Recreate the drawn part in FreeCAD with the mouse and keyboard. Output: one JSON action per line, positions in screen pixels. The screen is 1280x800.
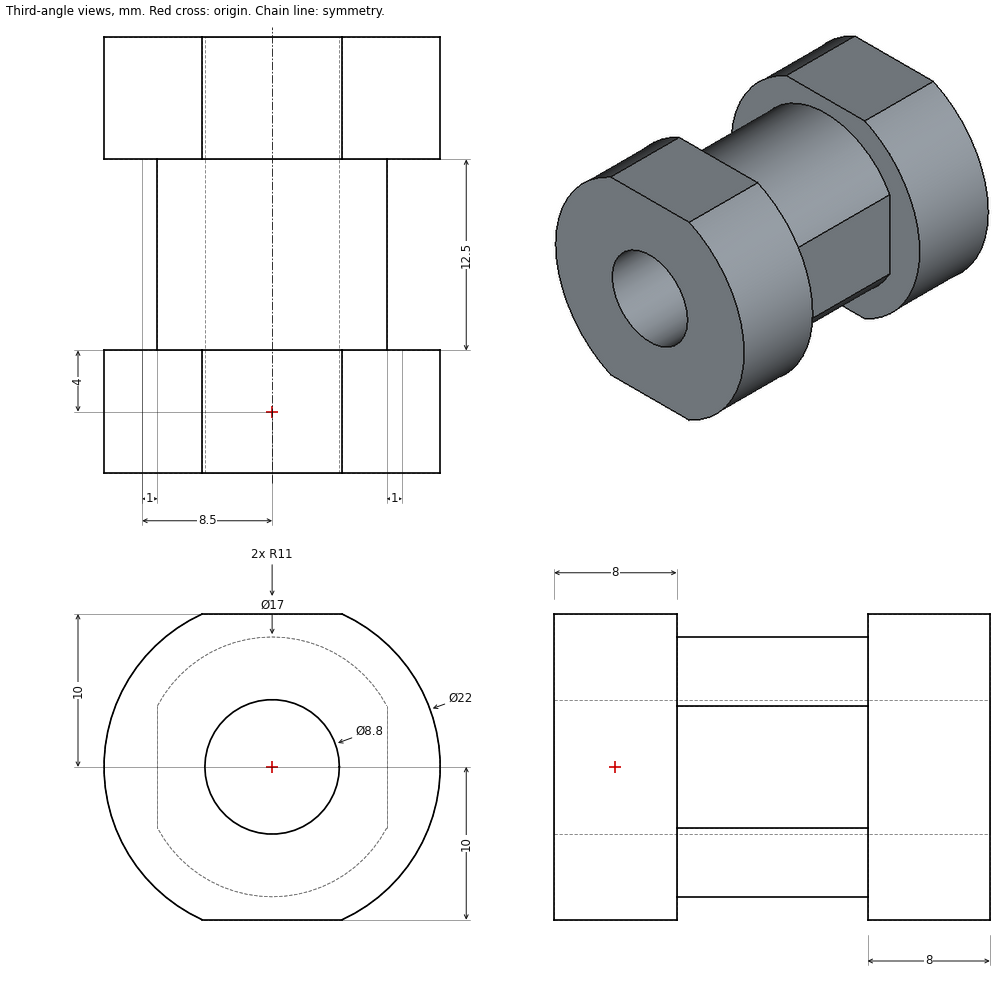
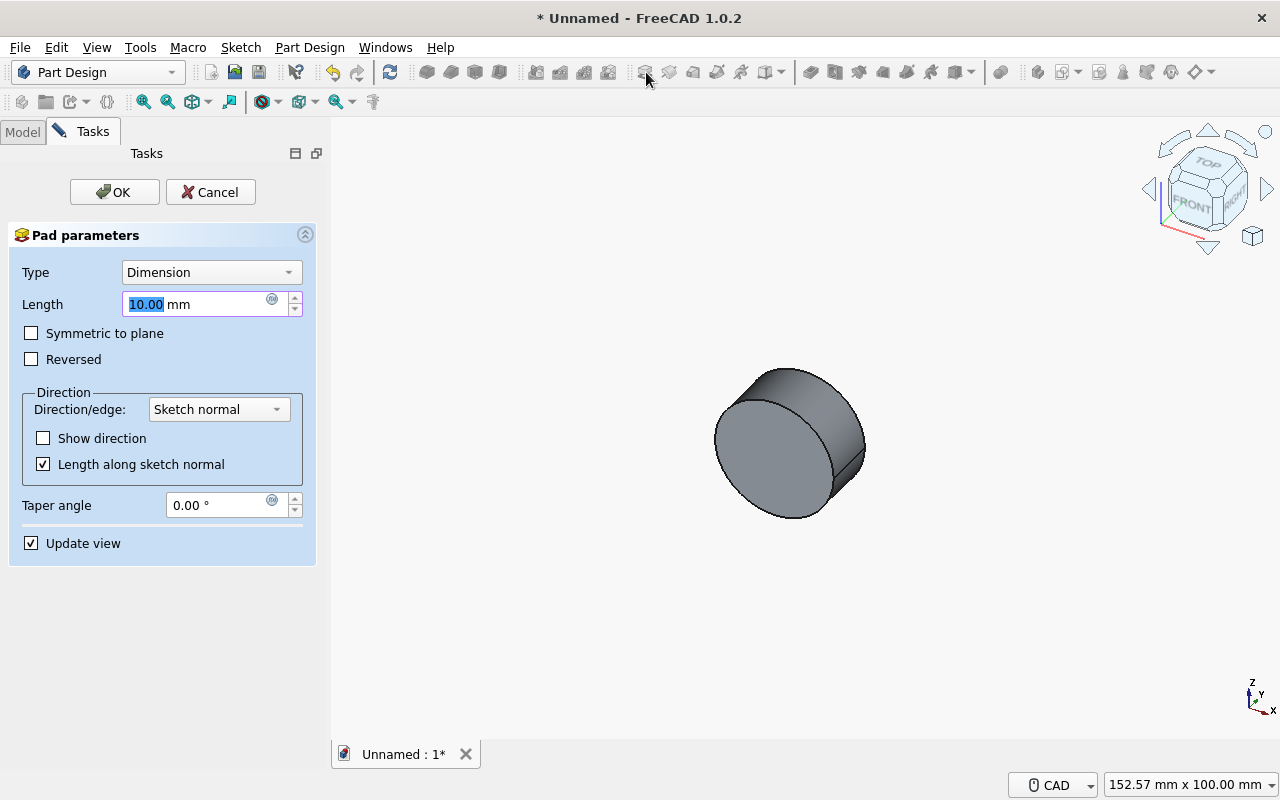
{"action": "type", "text": "8"}
{"action": "key", "text": "Tab"}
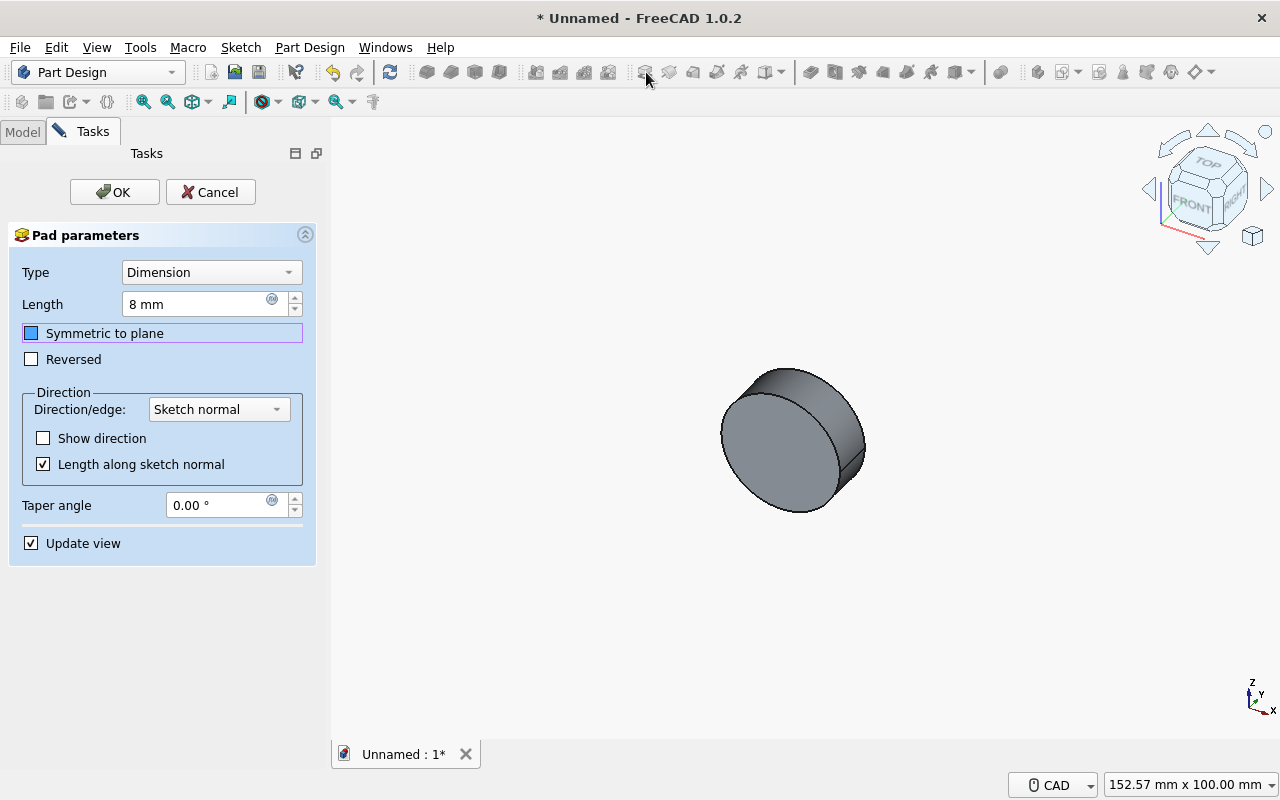
{"action": "left_click", "coordinate": [30, 333]}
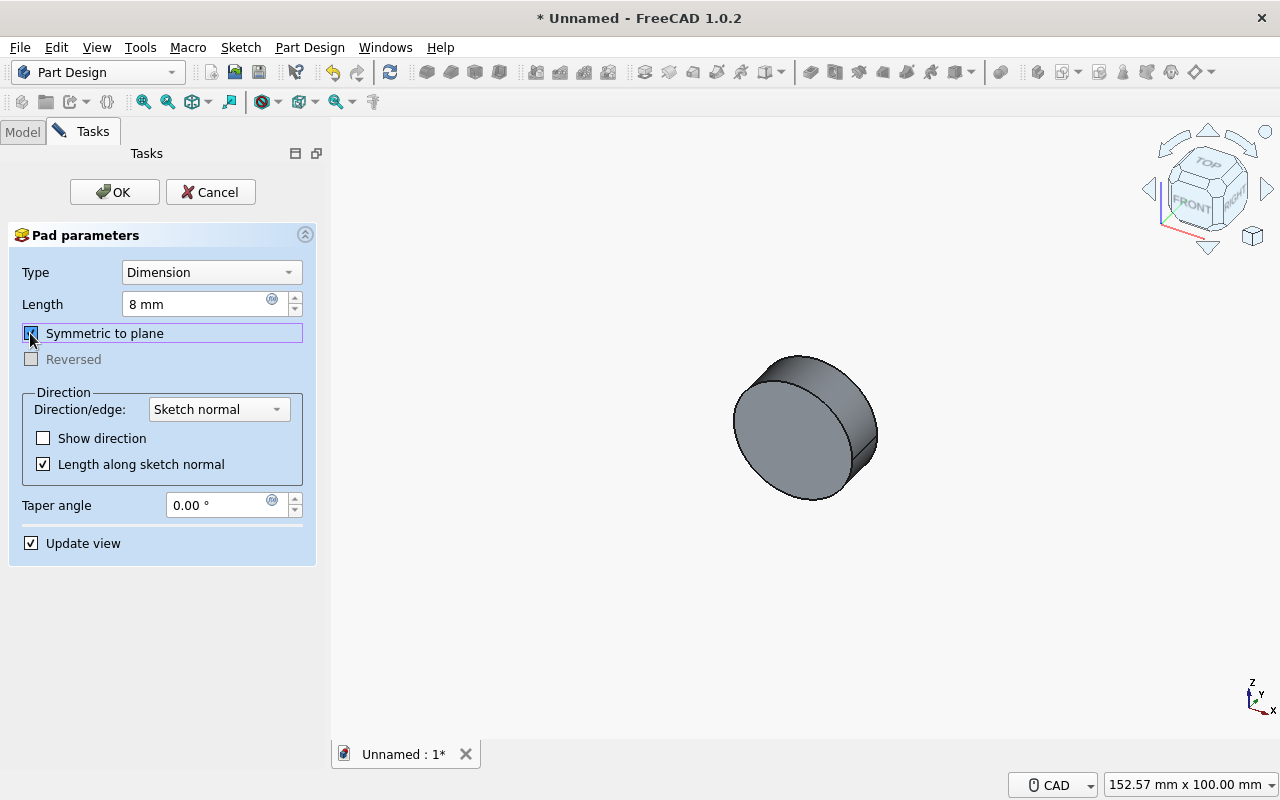
{"action": "left_click", "coordinate": [115, 192]}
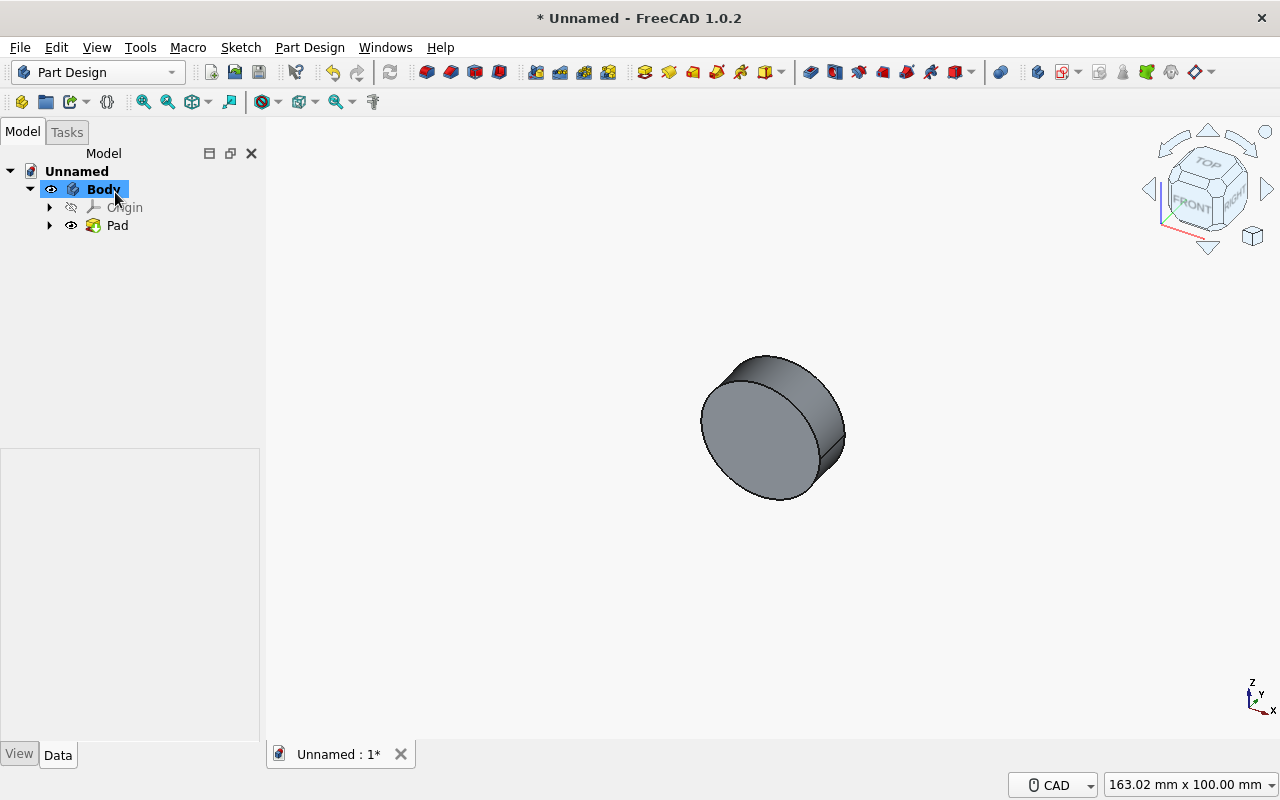
{"action": "left_click", "coordinate": [144, 102]}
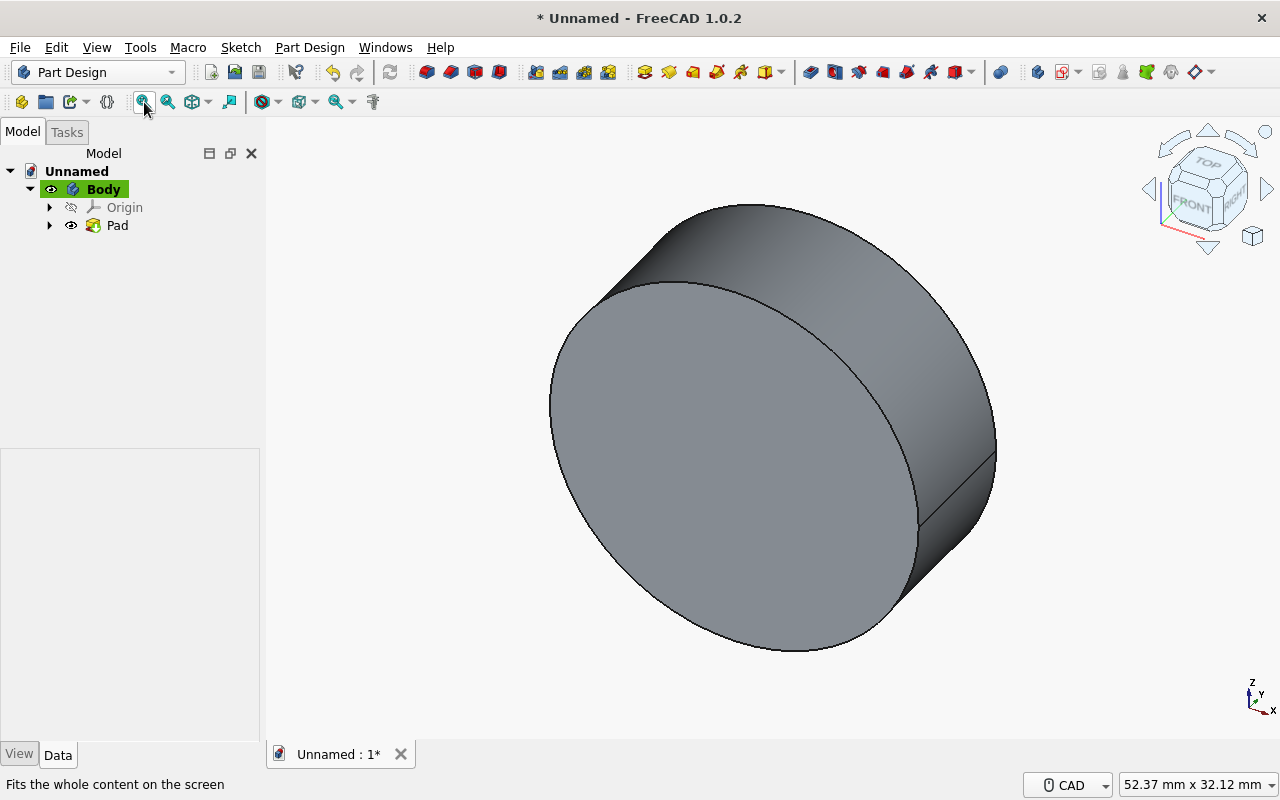
{"action": "key", "text": "4"}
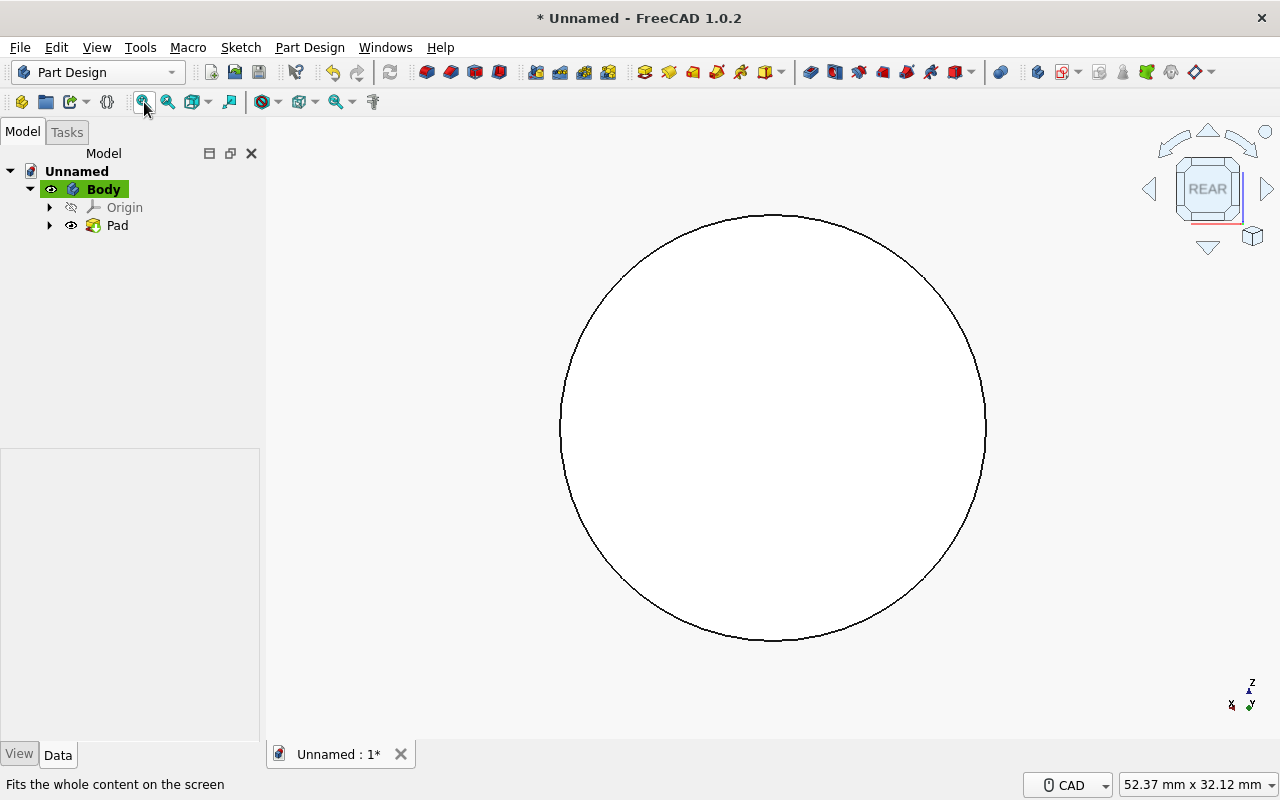
{"action": "left_click", "coordinate": [773, 427]}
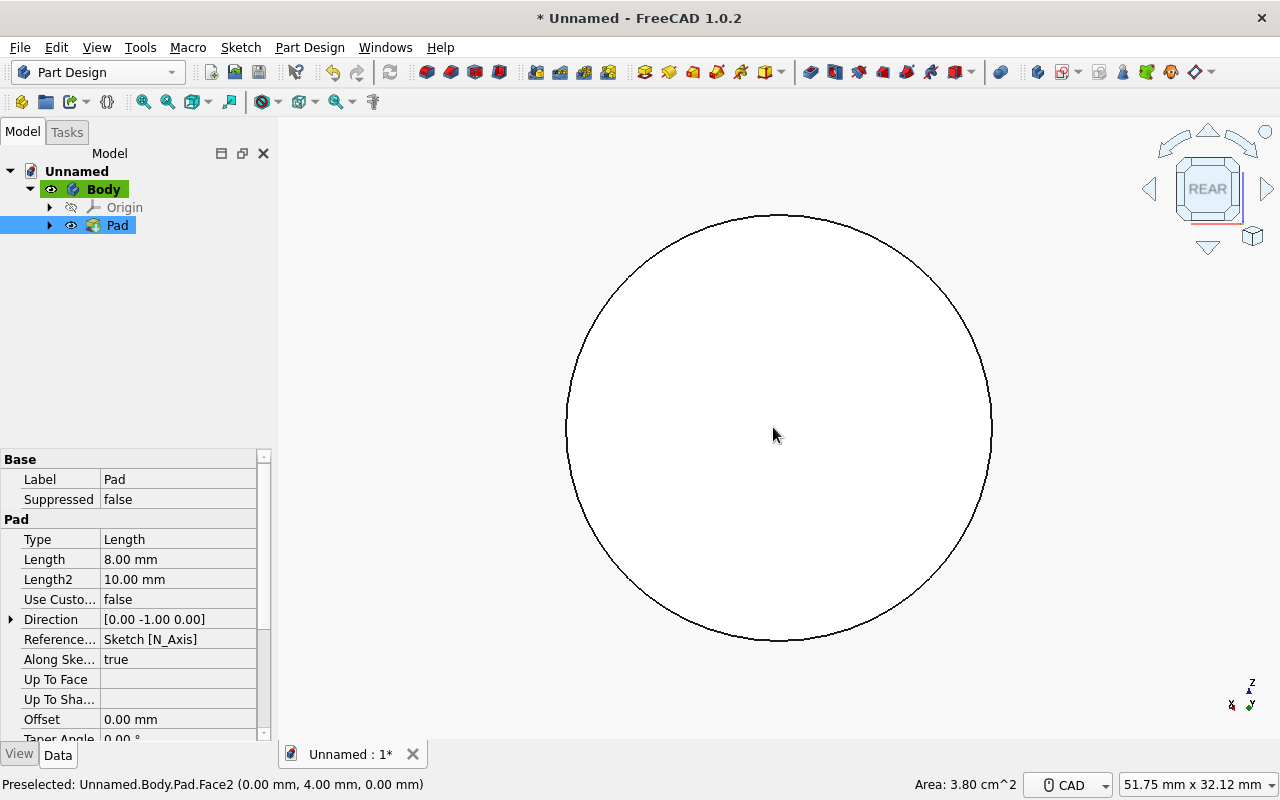
{"action": "left_click", "coordinate": [1062, 72]}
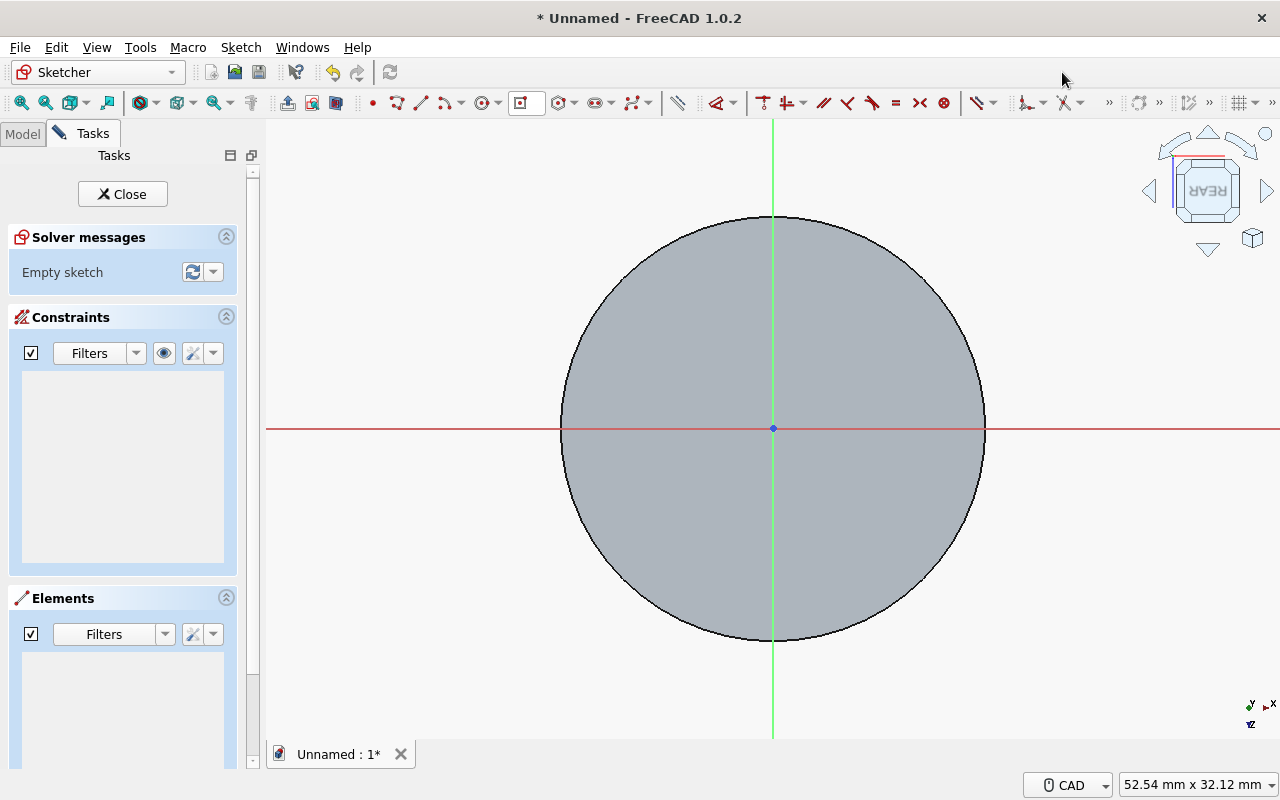
{"action": "left_click", "coordinate": [482, 104]}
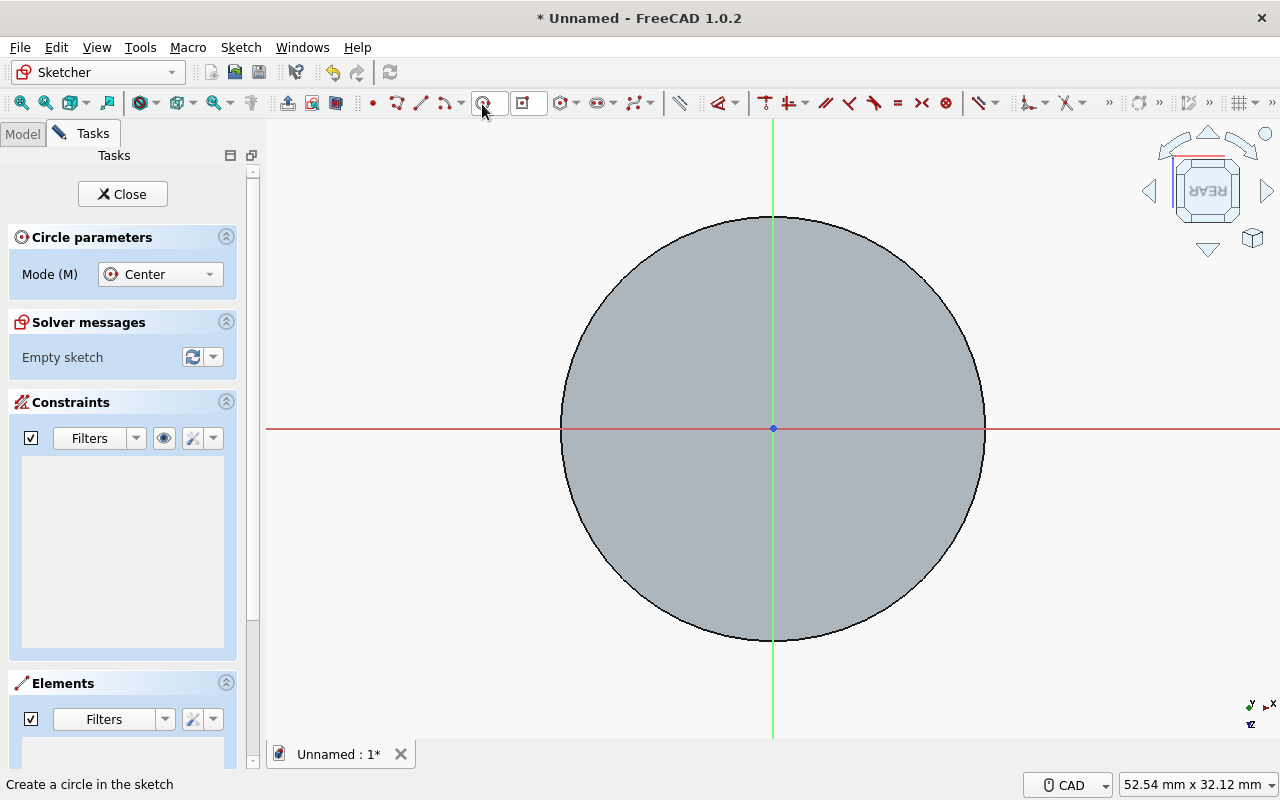
{"action": "left_click", "coordinate": [773, 429]}
{"action": "mouse_move", "coordinate": [889, 313]}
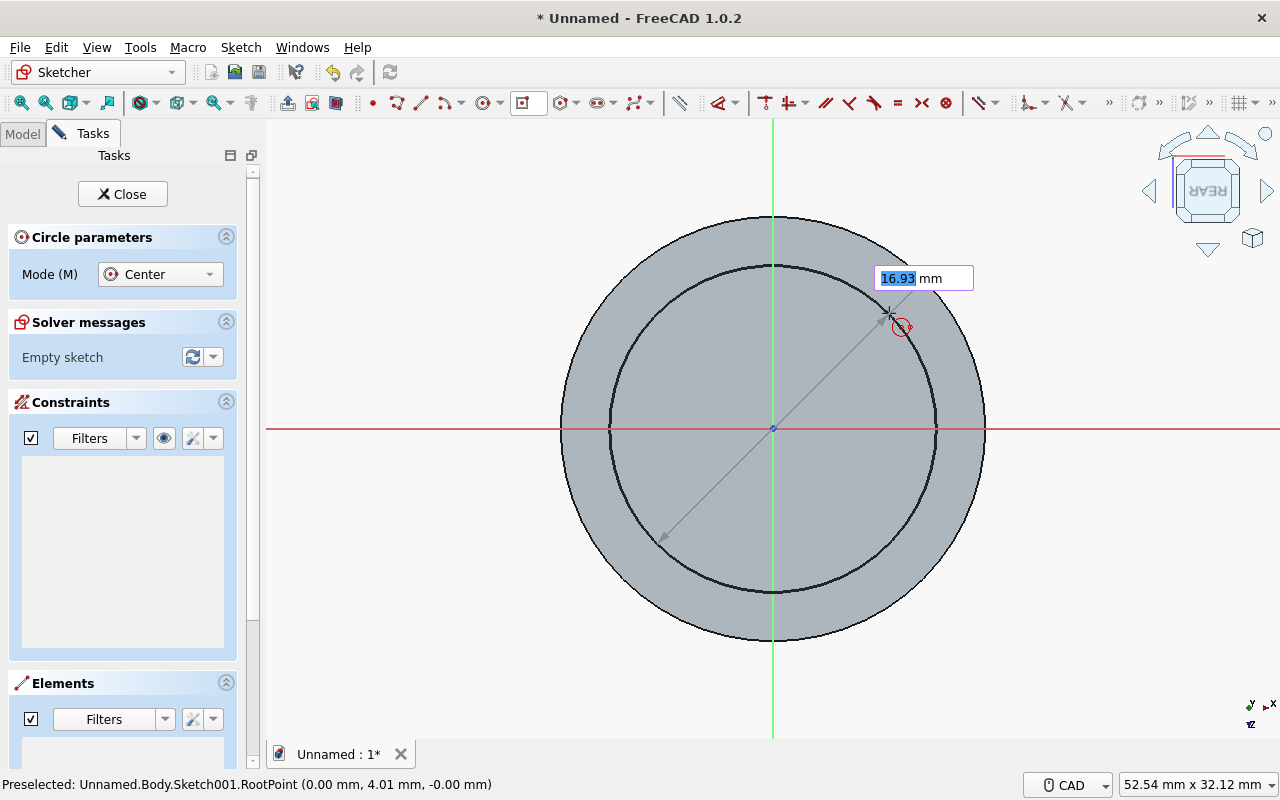
{"action": "type", "text": "17"}
{"action": "key", "text": "Return"}
{"action": "key", "text": "Escape"}